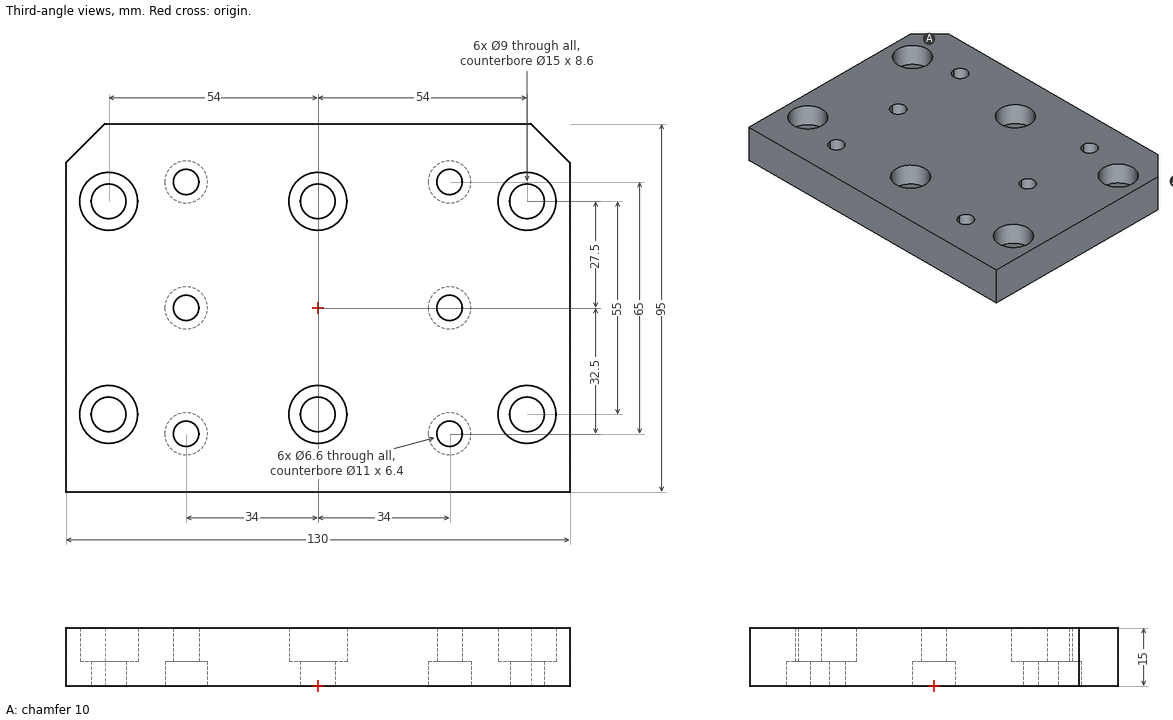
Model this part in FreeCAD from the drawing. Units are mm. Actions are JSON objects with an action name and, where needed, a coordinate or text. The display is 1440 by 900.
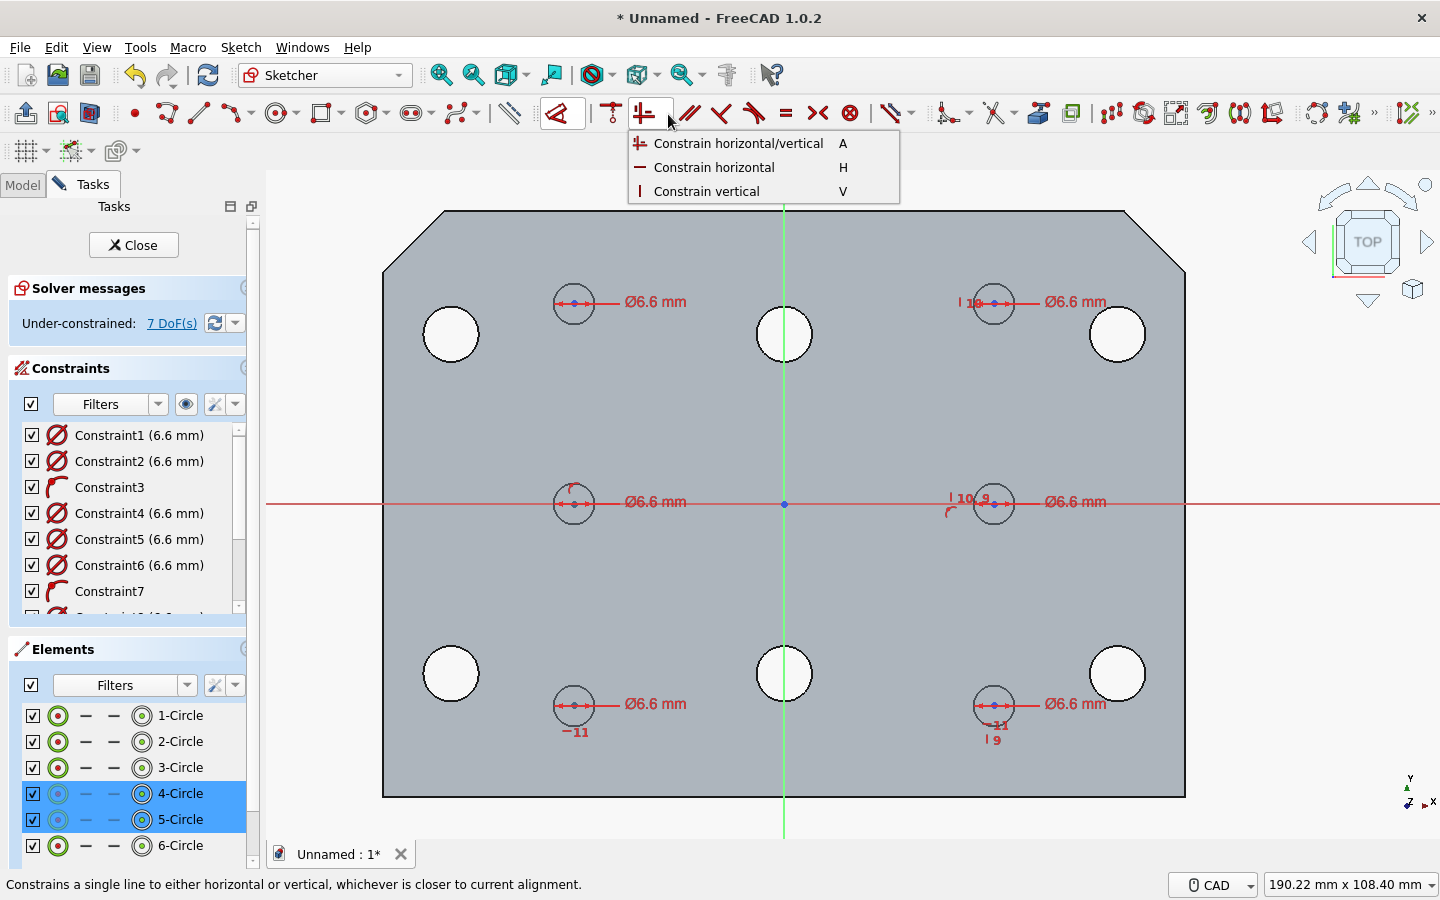
{"action": "left_click", "coordinate": [764, 191]}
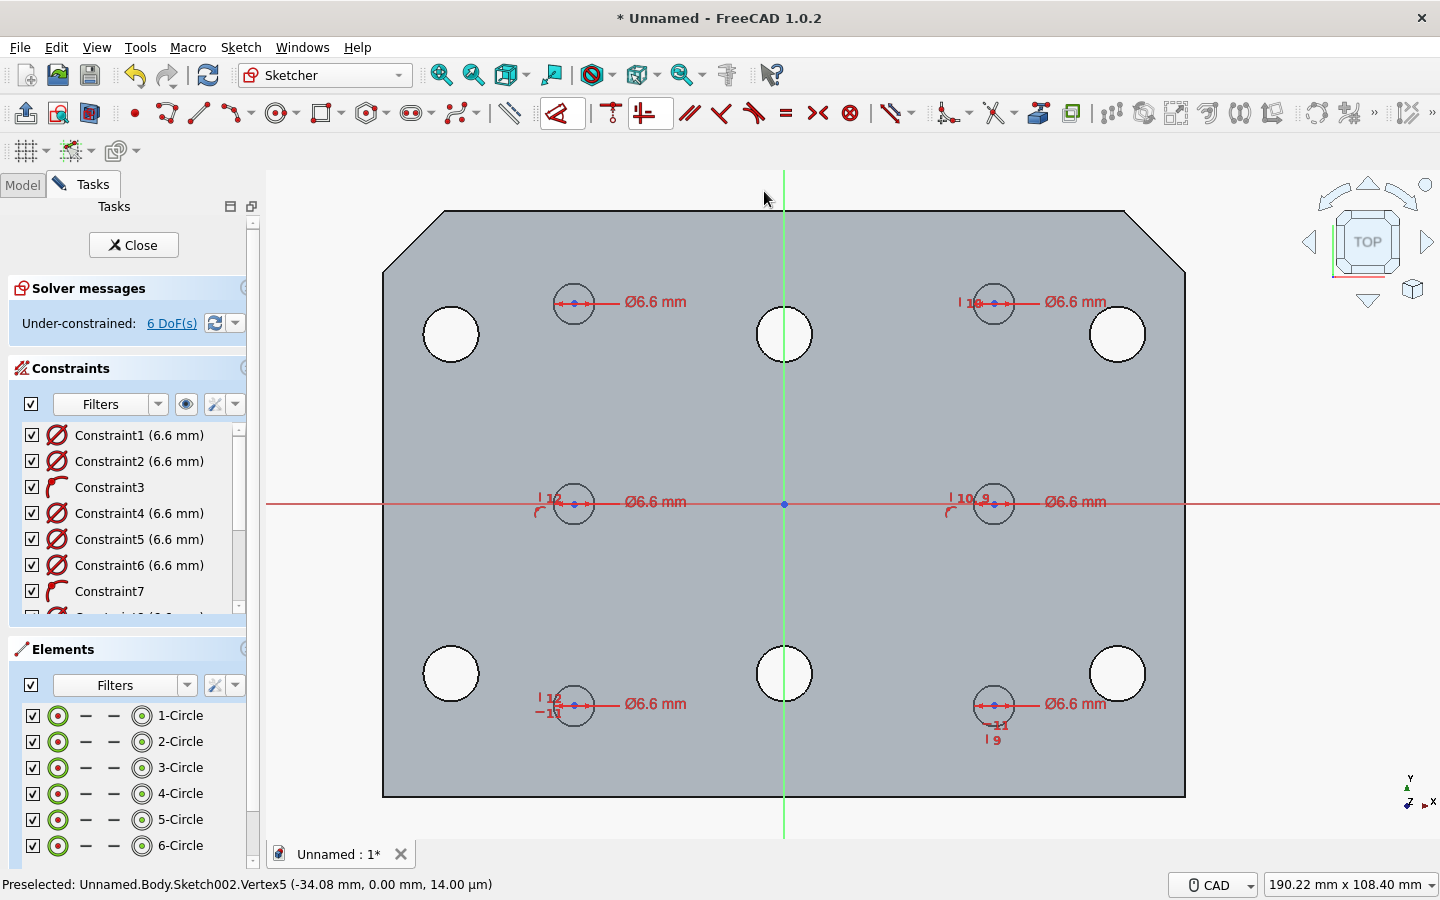
{"action": "left_click", "coordinate": [574, 504]}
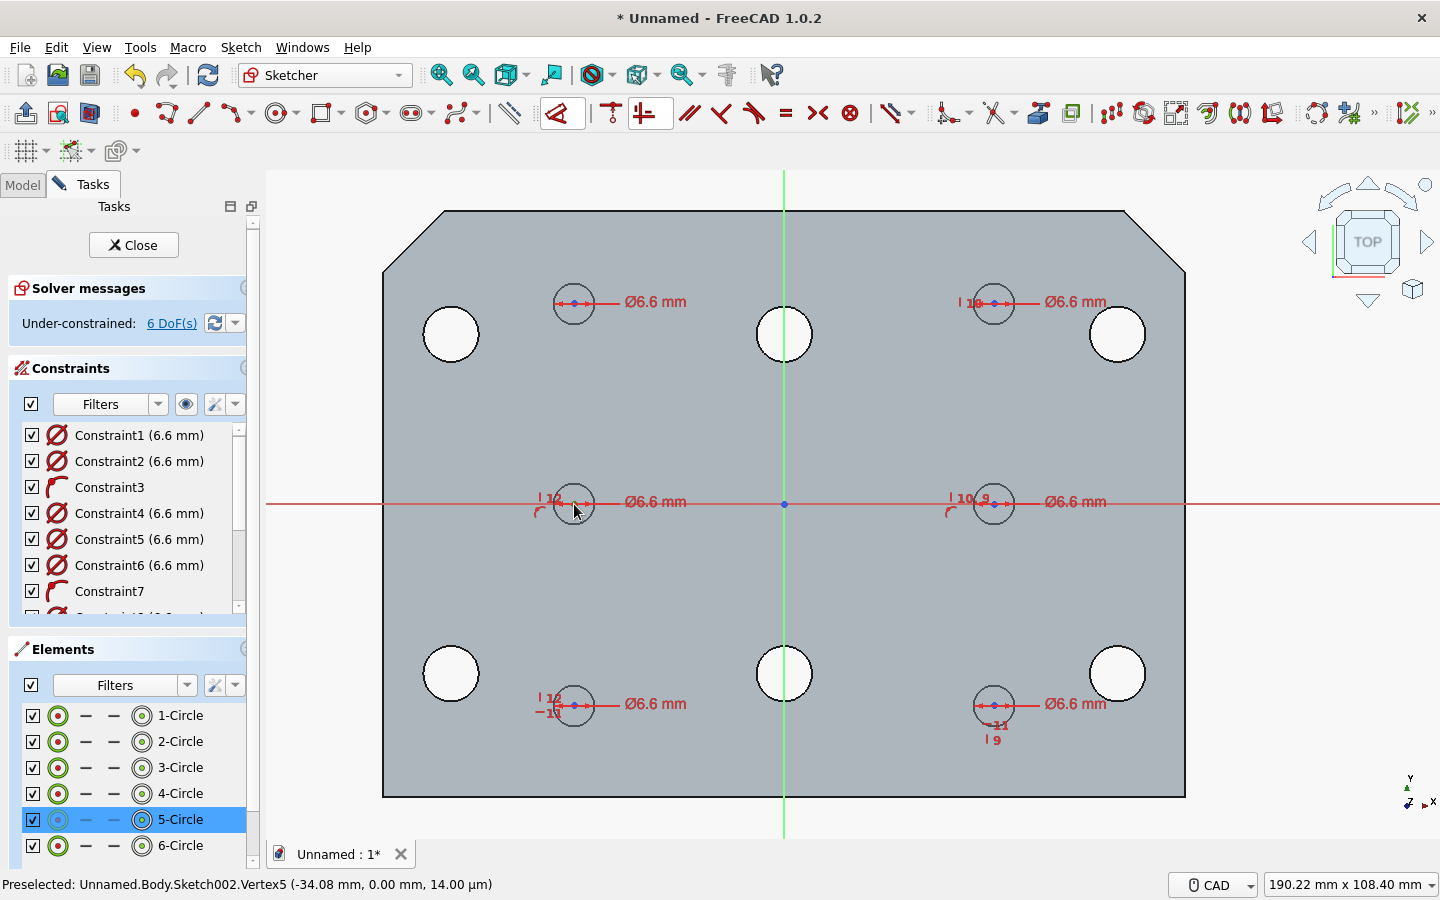
{"action": "left_click", "coordinate": [574, 304]}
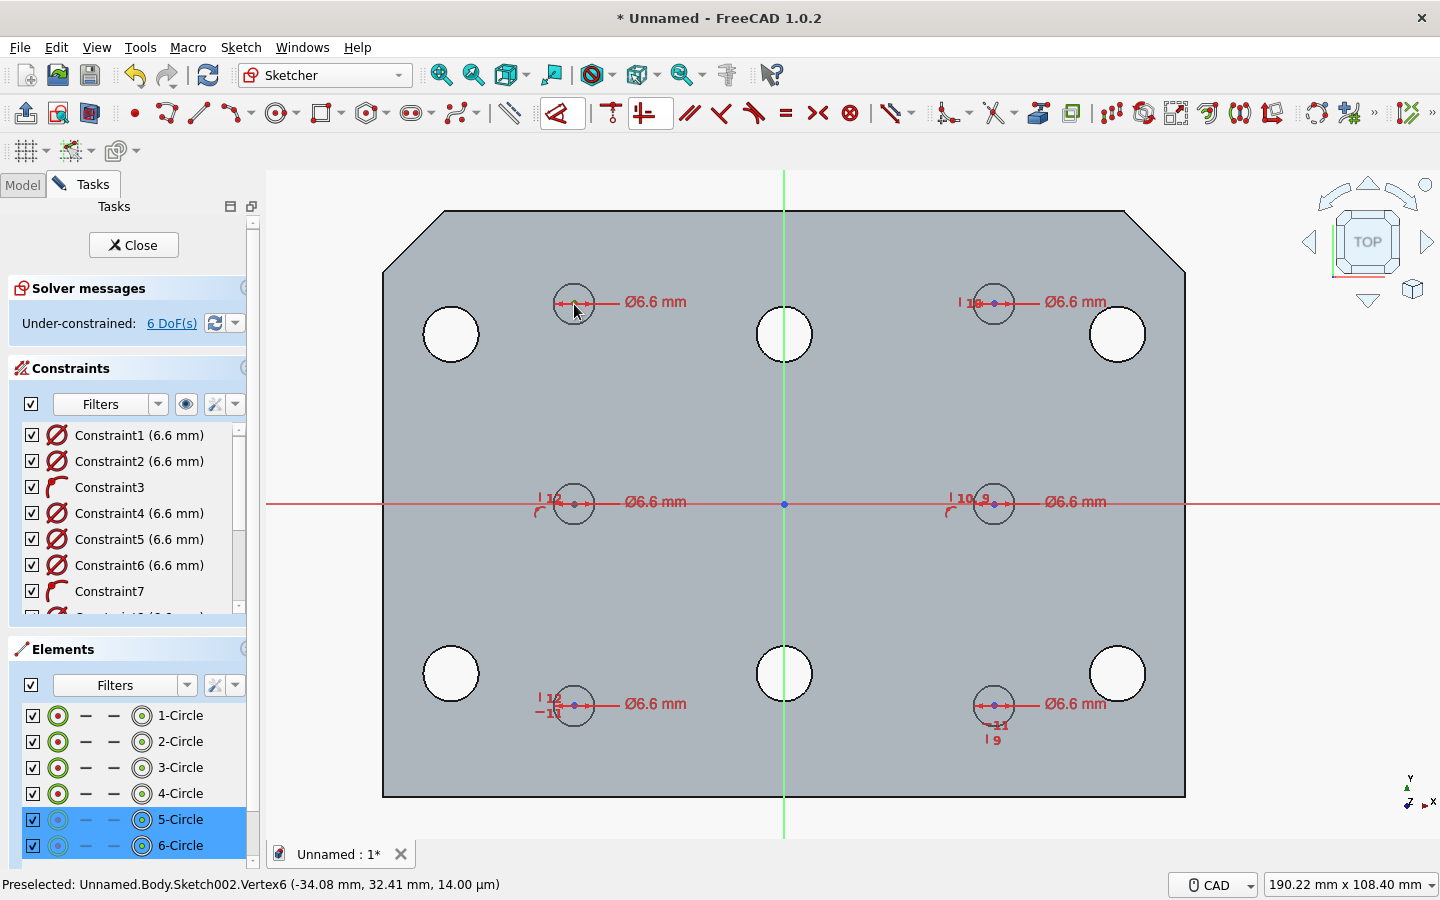
{"action": "left_click", "coordinate": [668, 114]}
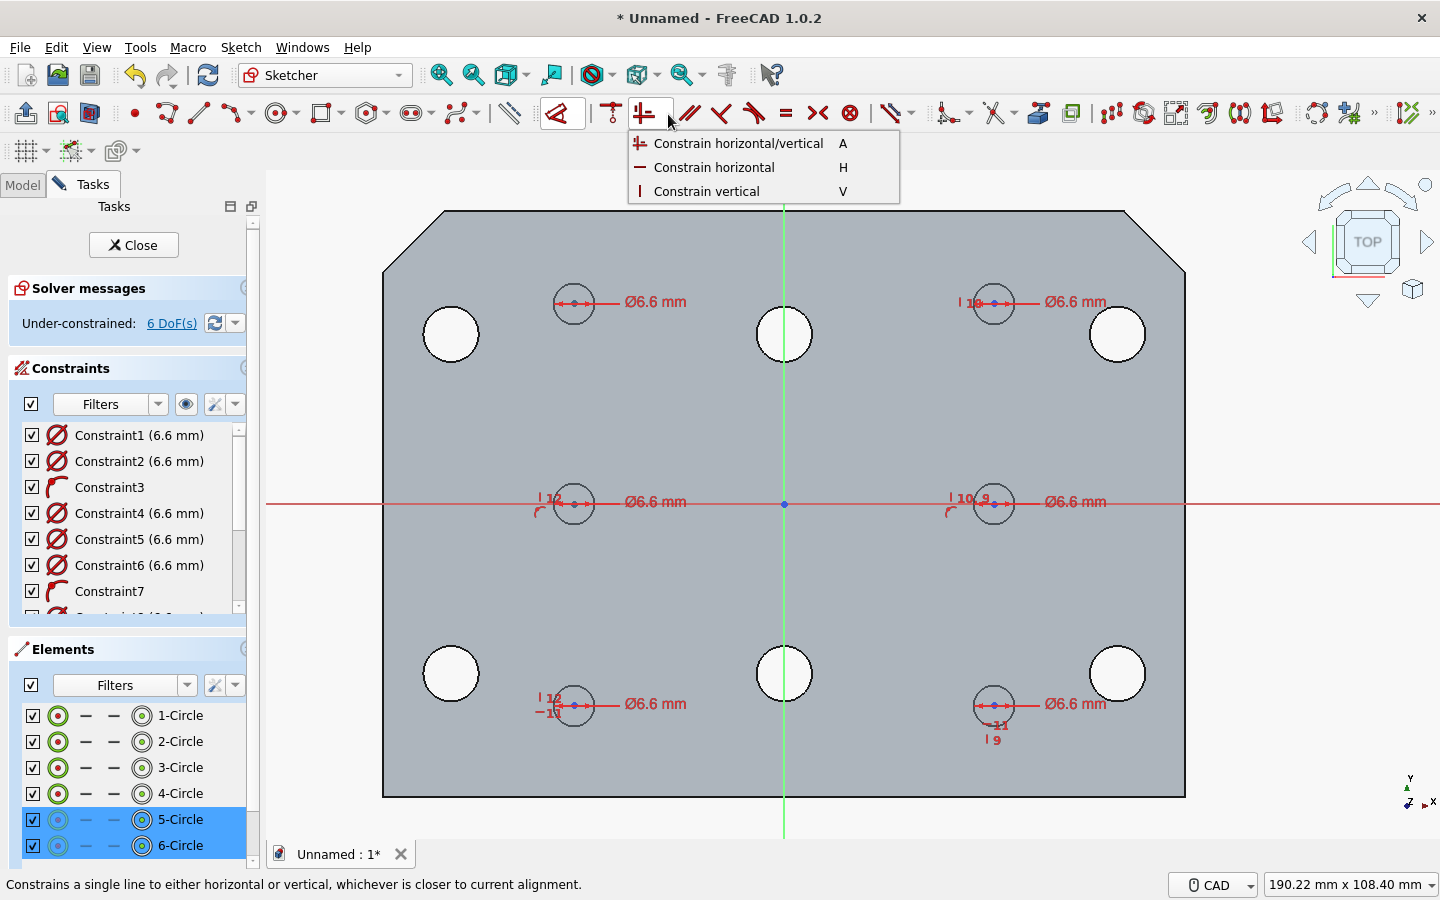
{"action": "left_click", "coordinate": [764, 191]}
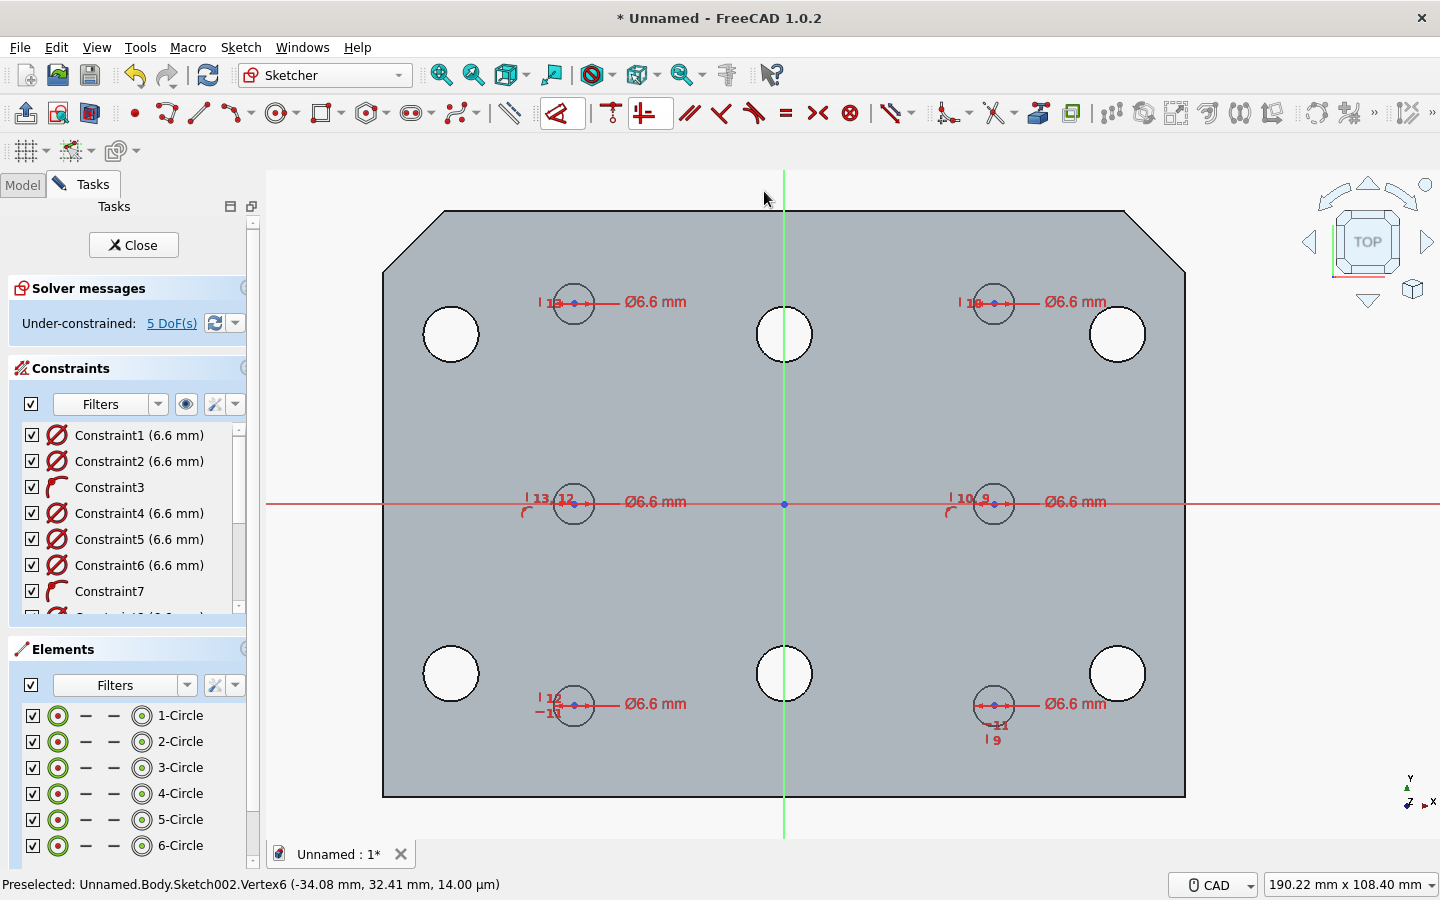
{"action": "left_click", "coordinate": [994, 304]}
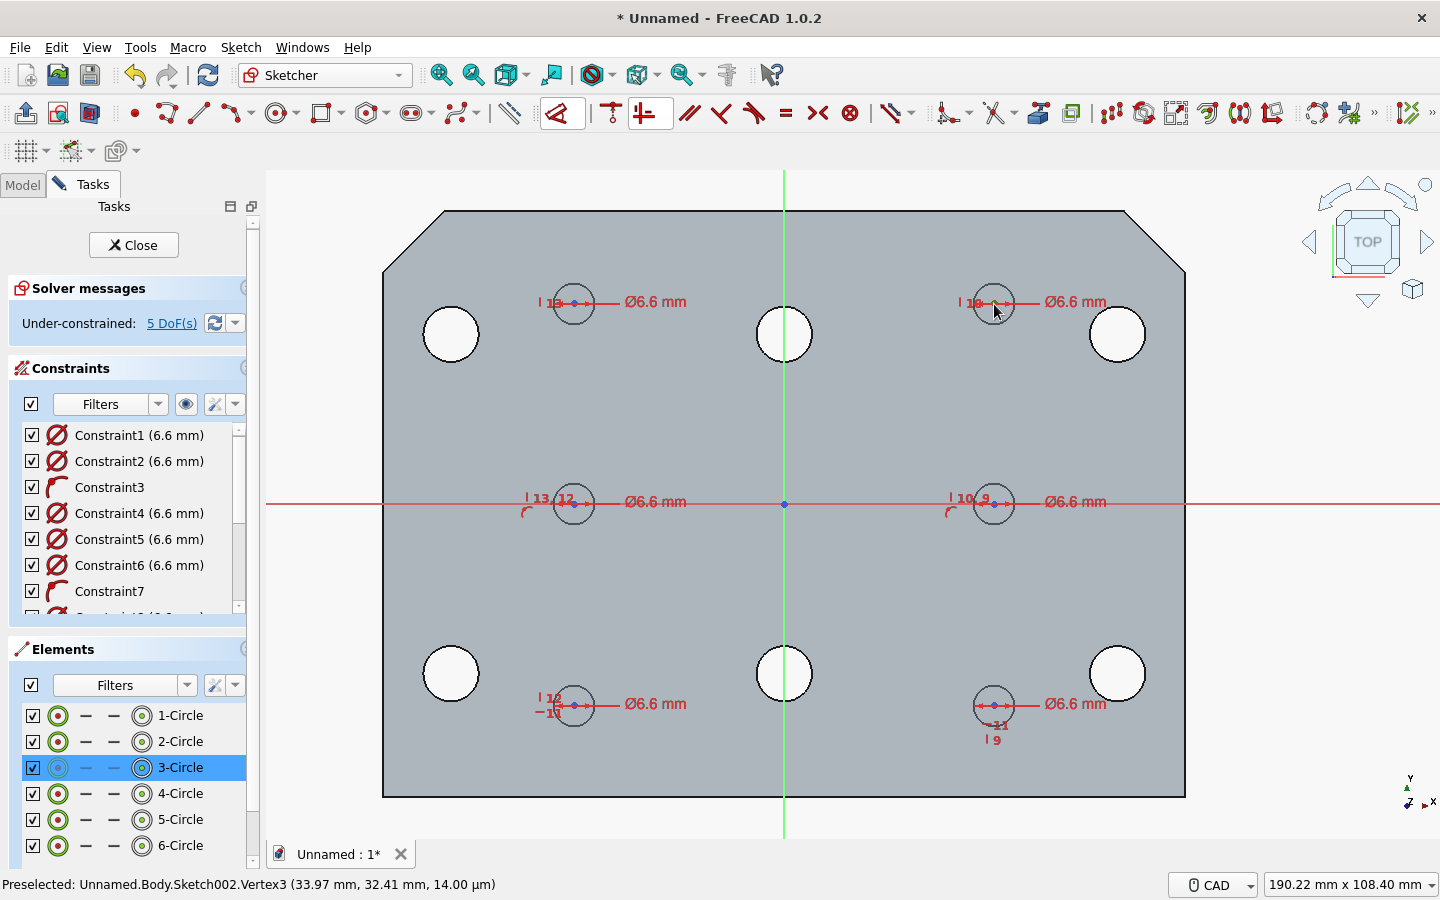
{"action": "left_click", "coordinate": [574, 304]}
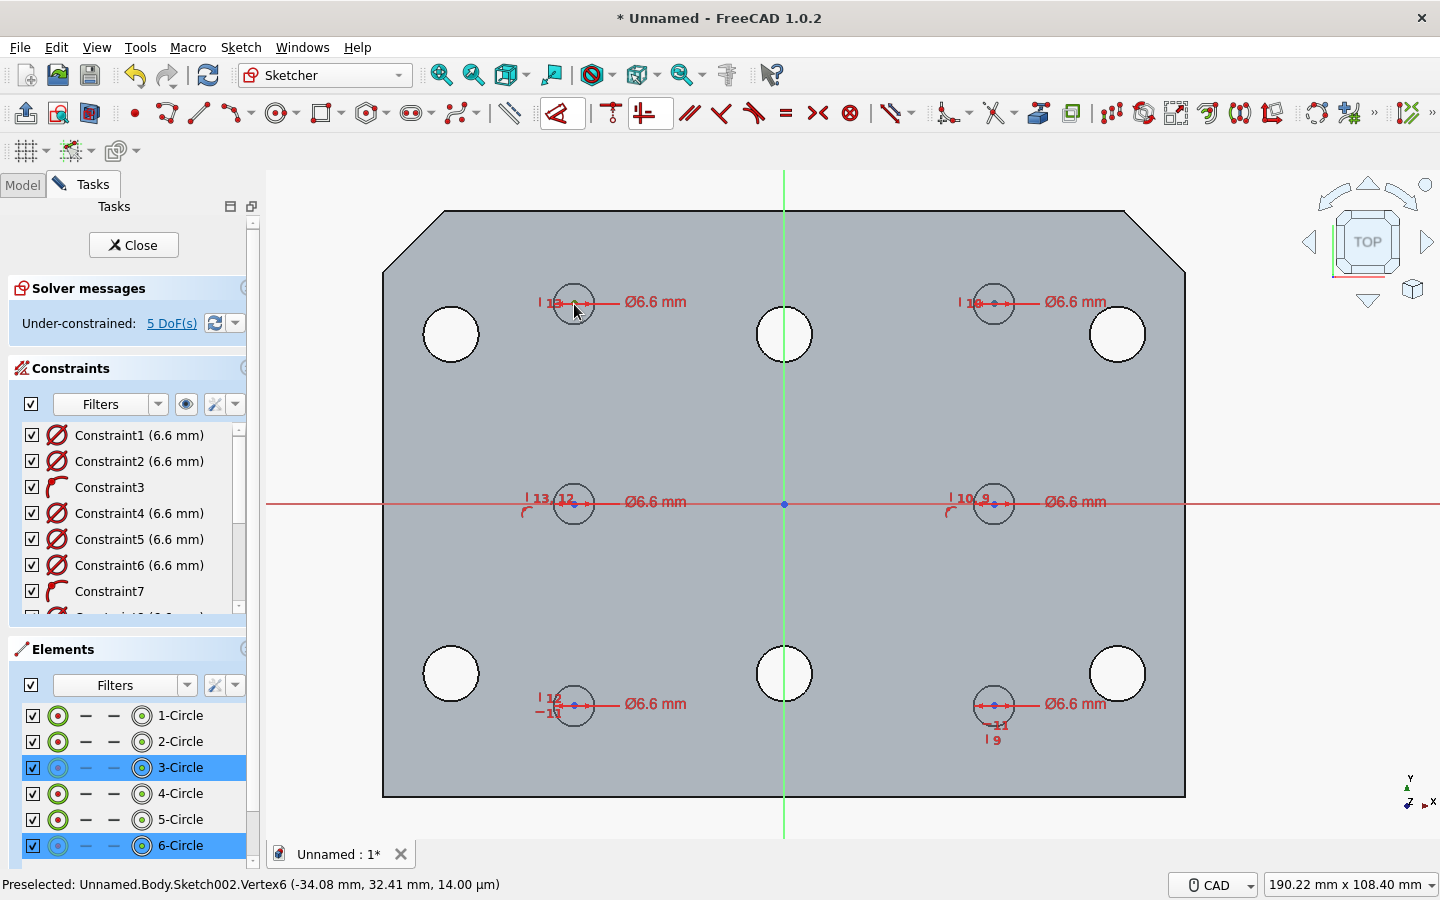
{"action": "key", "text": "h"}